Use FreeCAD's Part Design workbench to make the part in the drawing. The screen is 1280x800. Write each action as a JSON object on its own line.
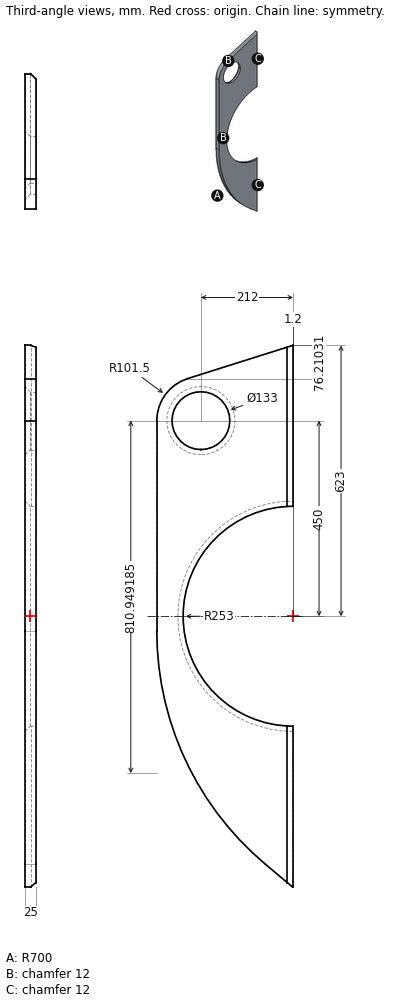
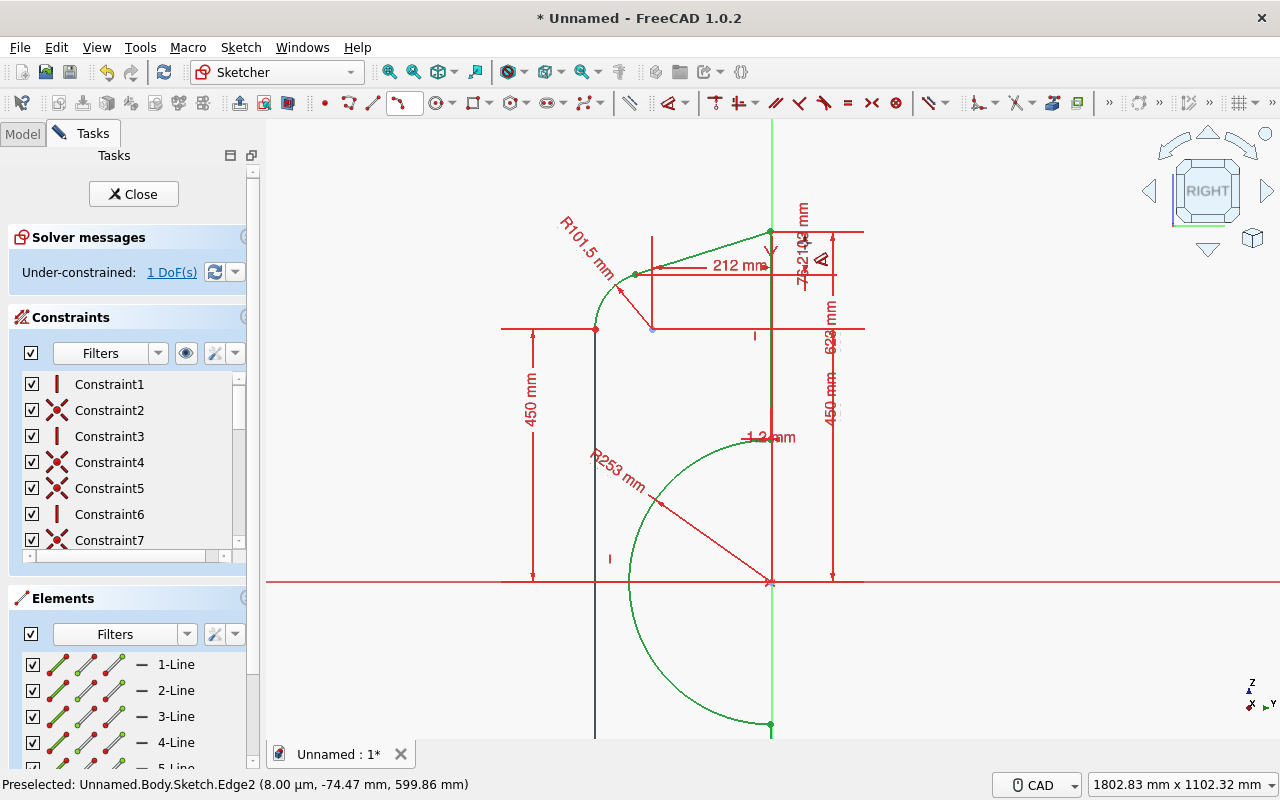
{"action": "left_click", "coordinate": [595, 467]}
{"action": "left_click", "coordinate": [561, 520]}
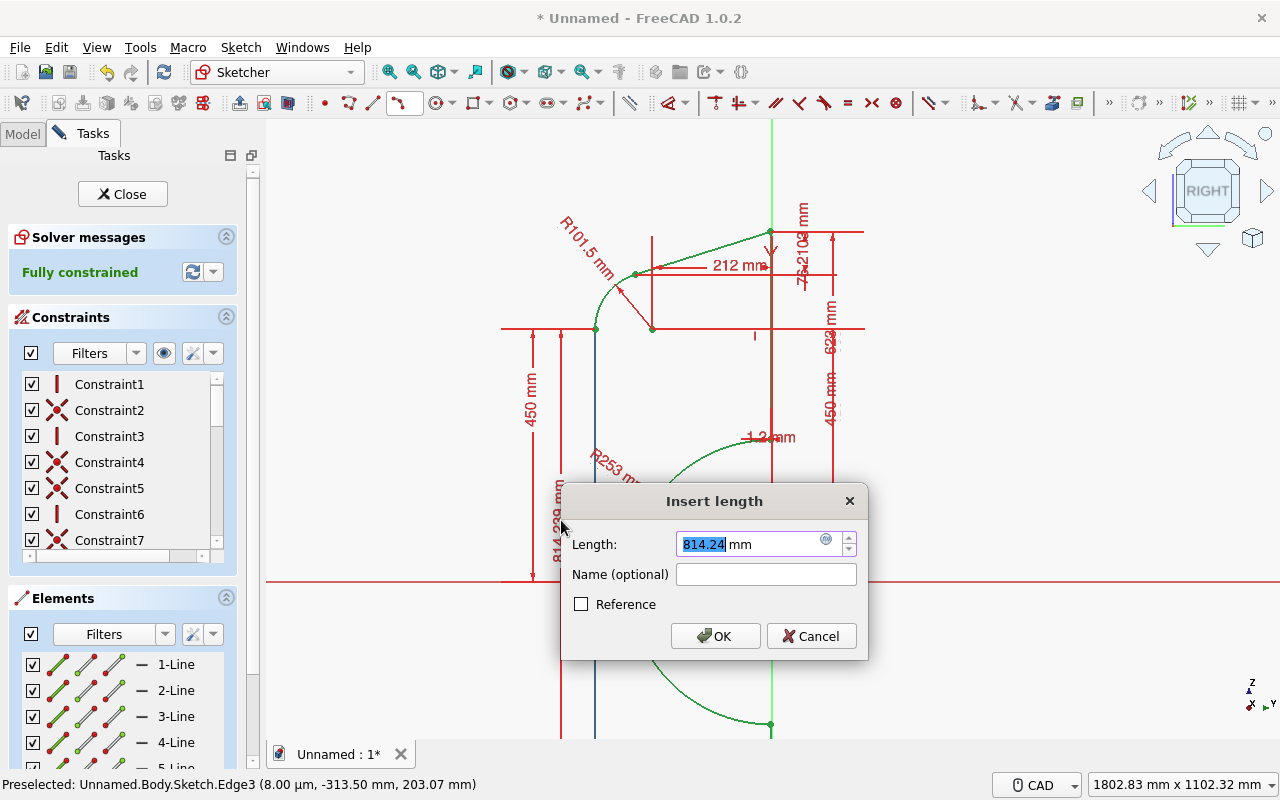
{"action": "type", "text": "810.949185"}
{"action": "key", "text": "Return"}
{"action": "key", "text": "Escape"}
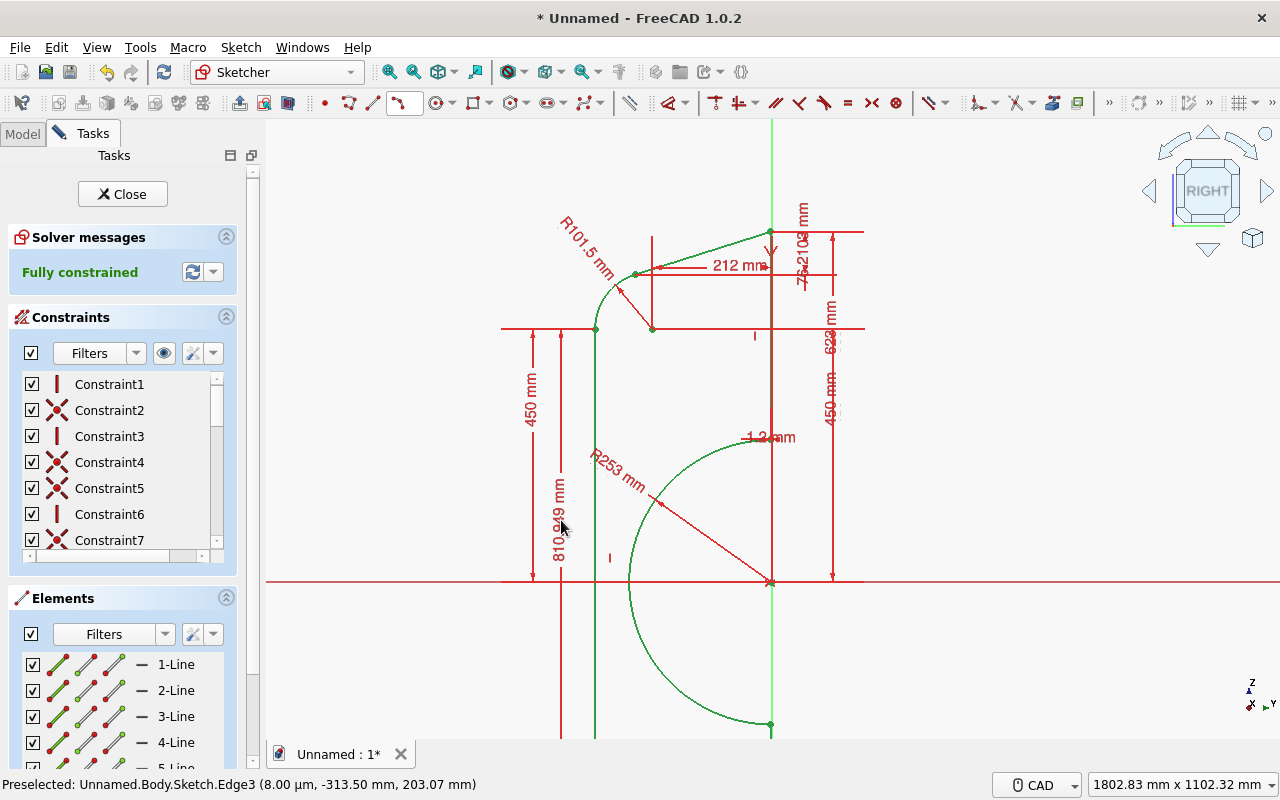
{"action": "left_click", "coordinate": [123, 194]}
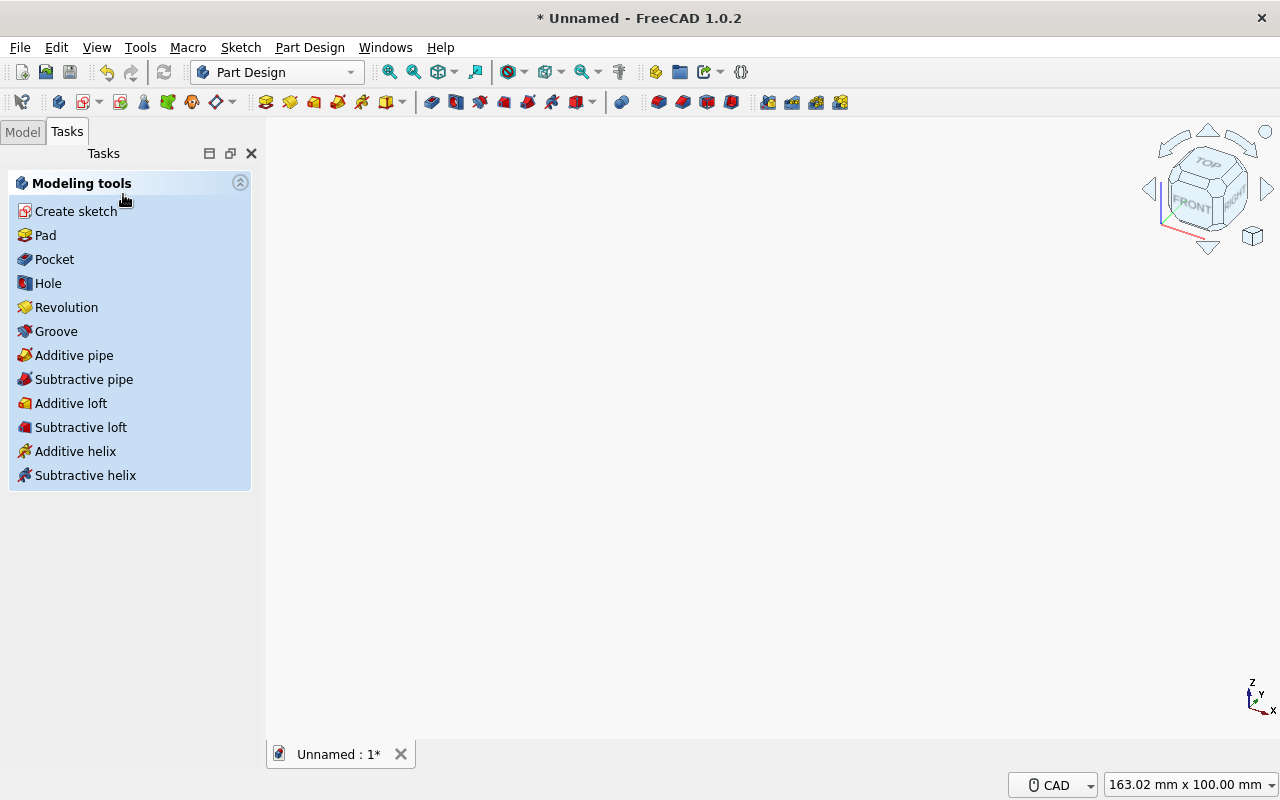
{"action": "left_click", "coordinate": [266, 102]}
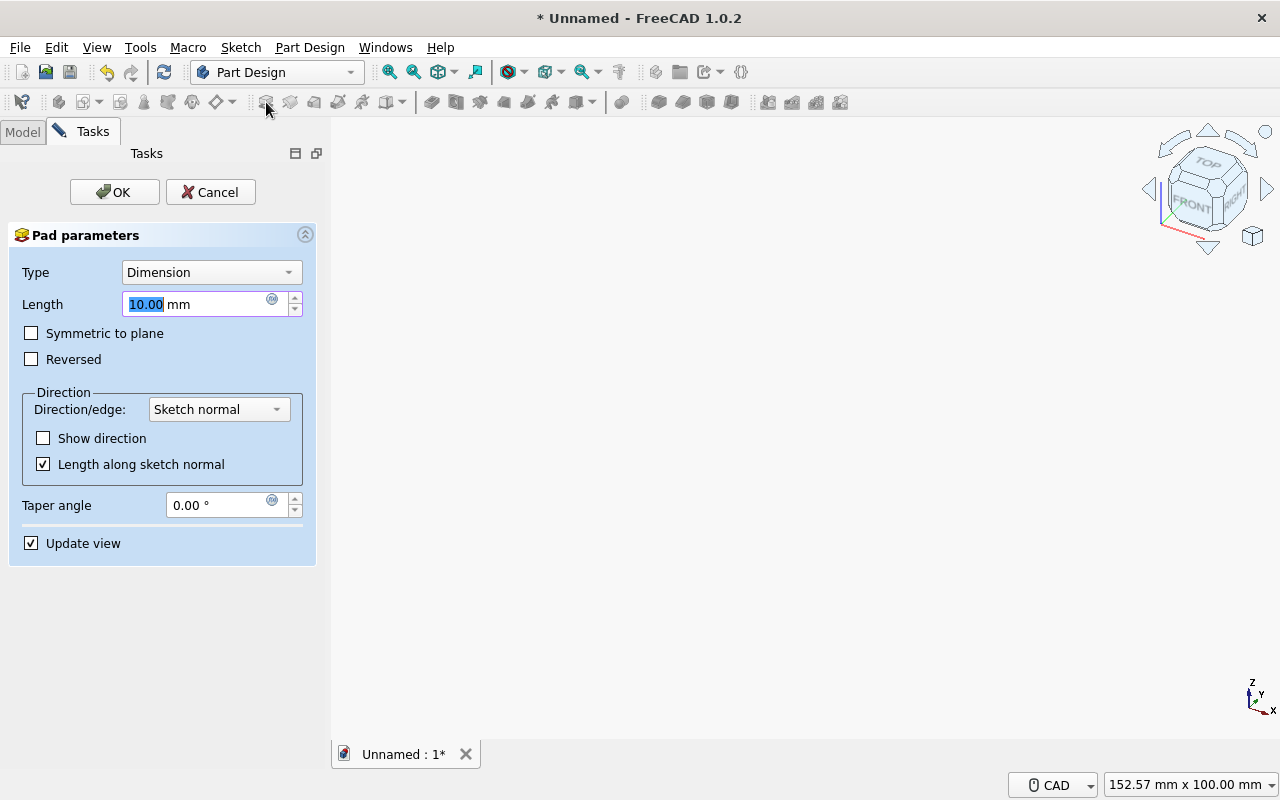
{"action": "type", "text": "25"}
{"action": "key", "text": "Tab"}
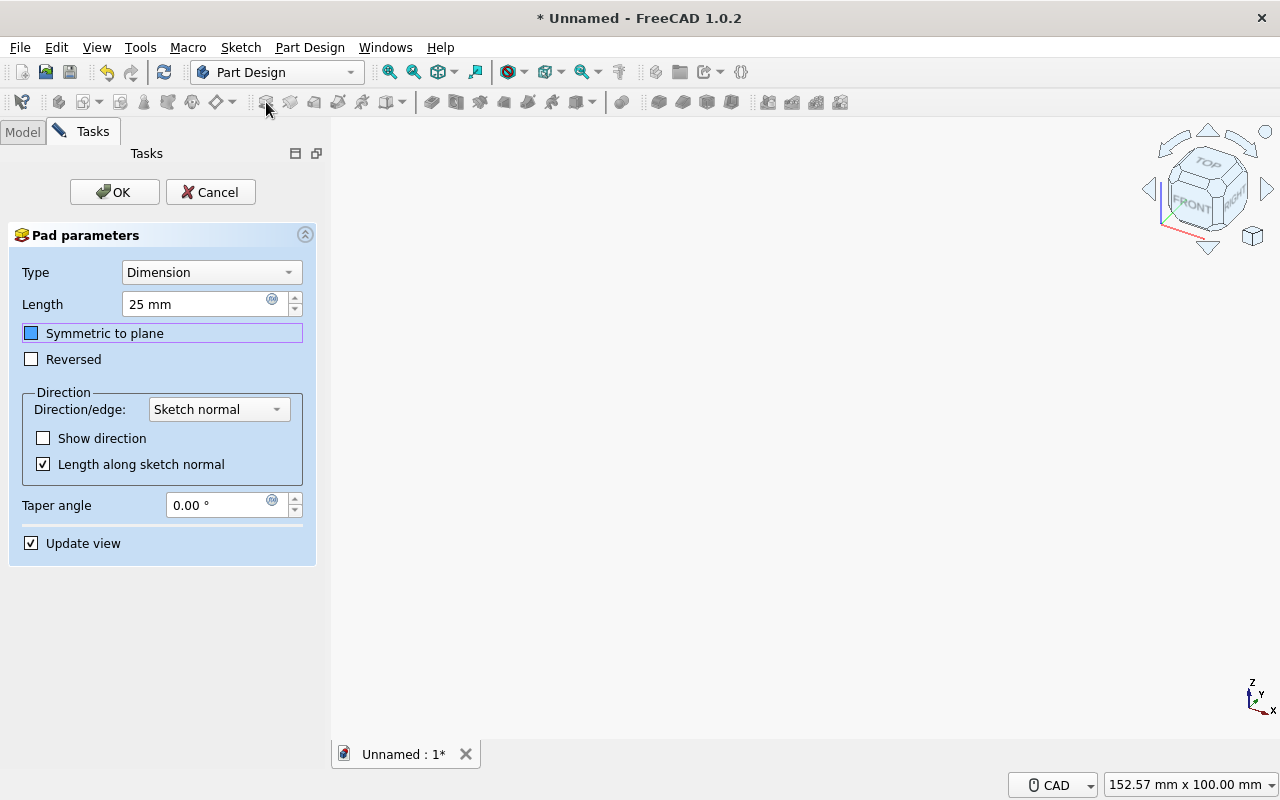
{"action": "left_click", "coordinate": [30, 333]}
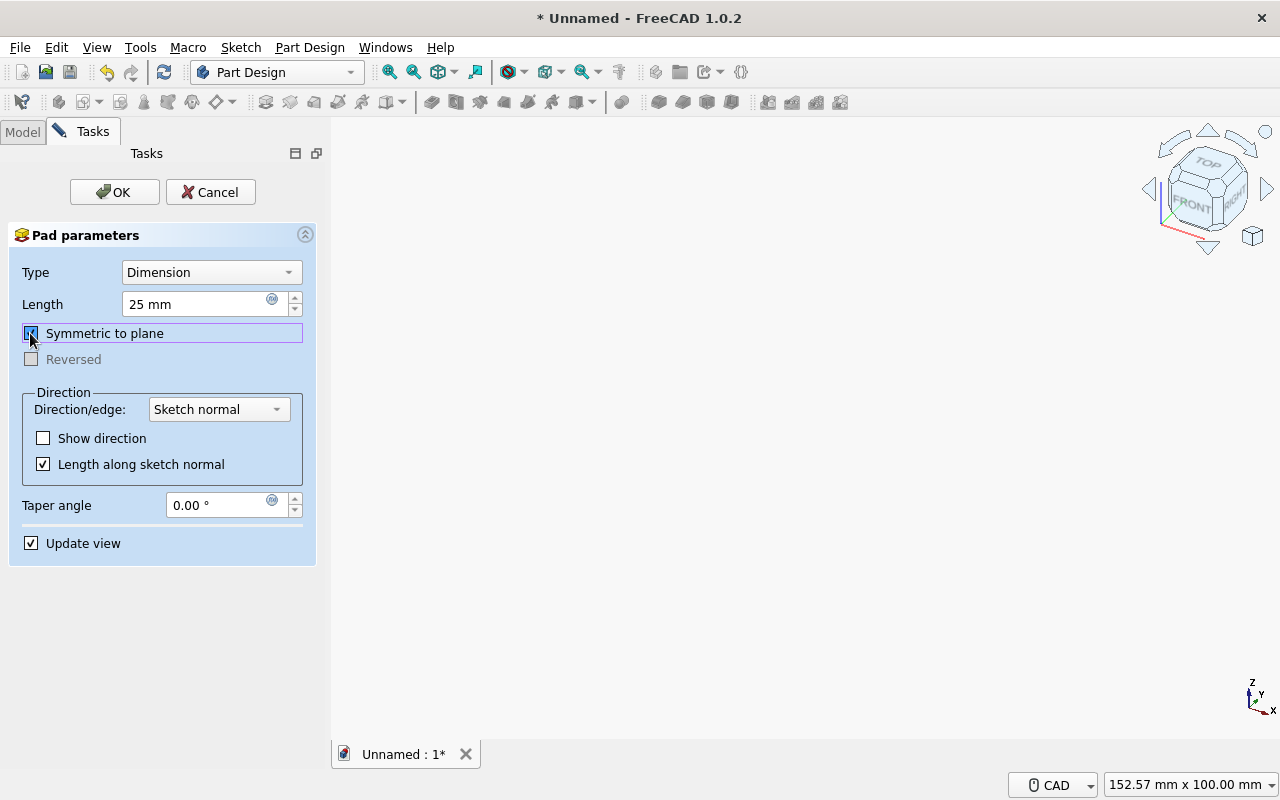
{"action": "left_click", "coordinate": [115, 192]}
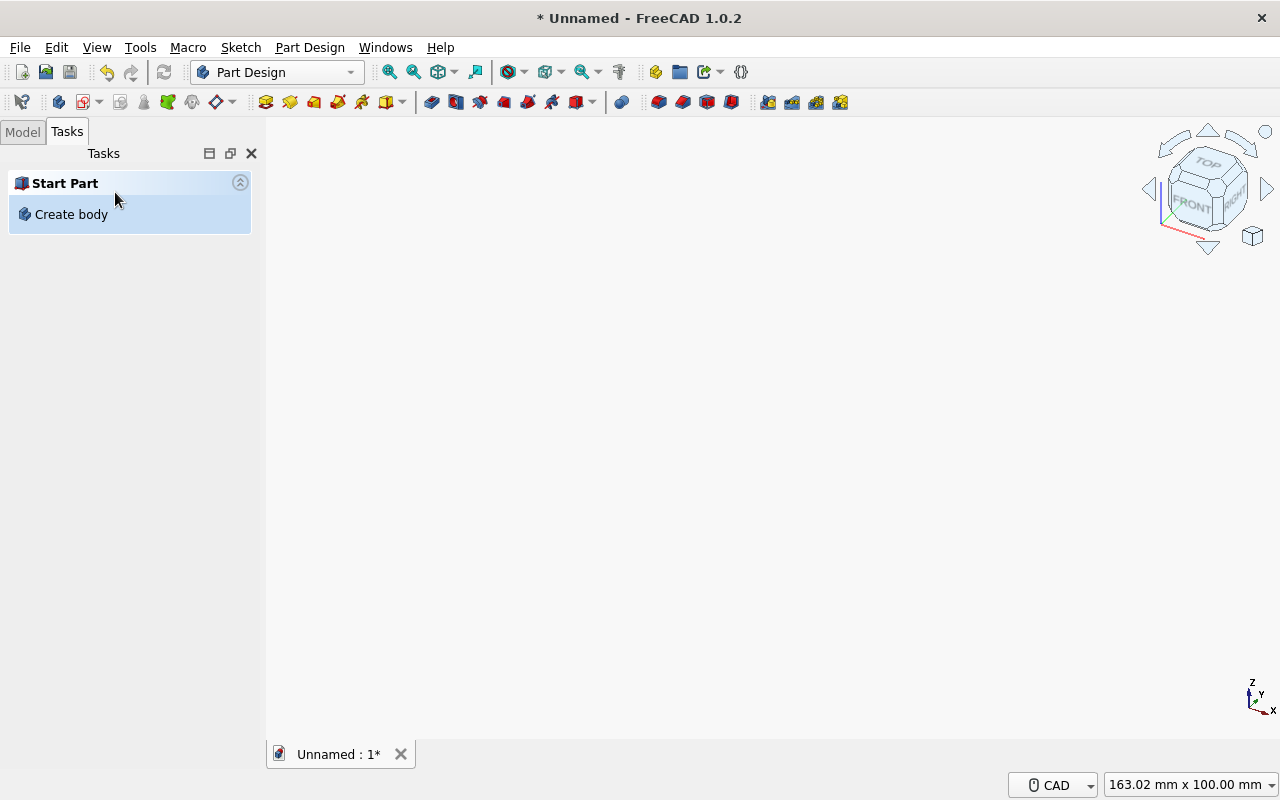
{"action": "left_click", "coordinate": [390, 72]}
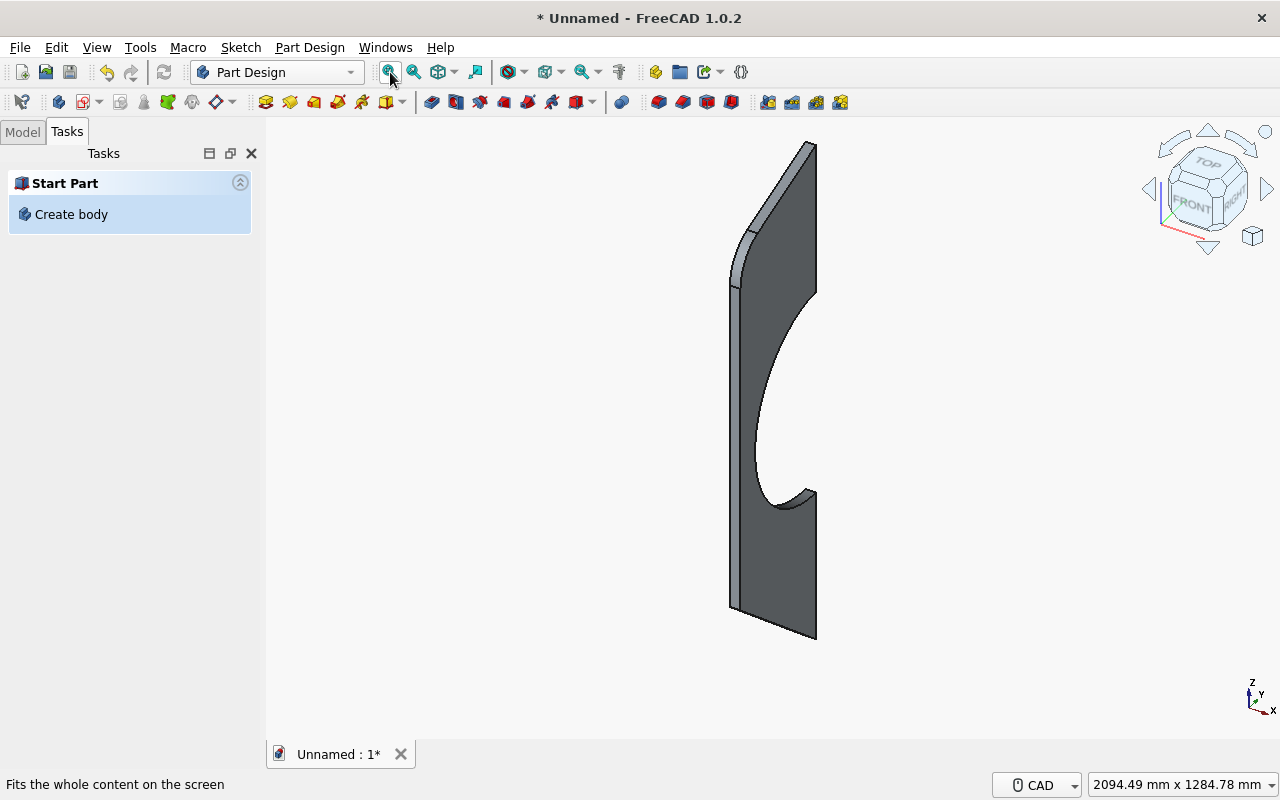
{"action": "left_click", "coordinate": [84, 102]}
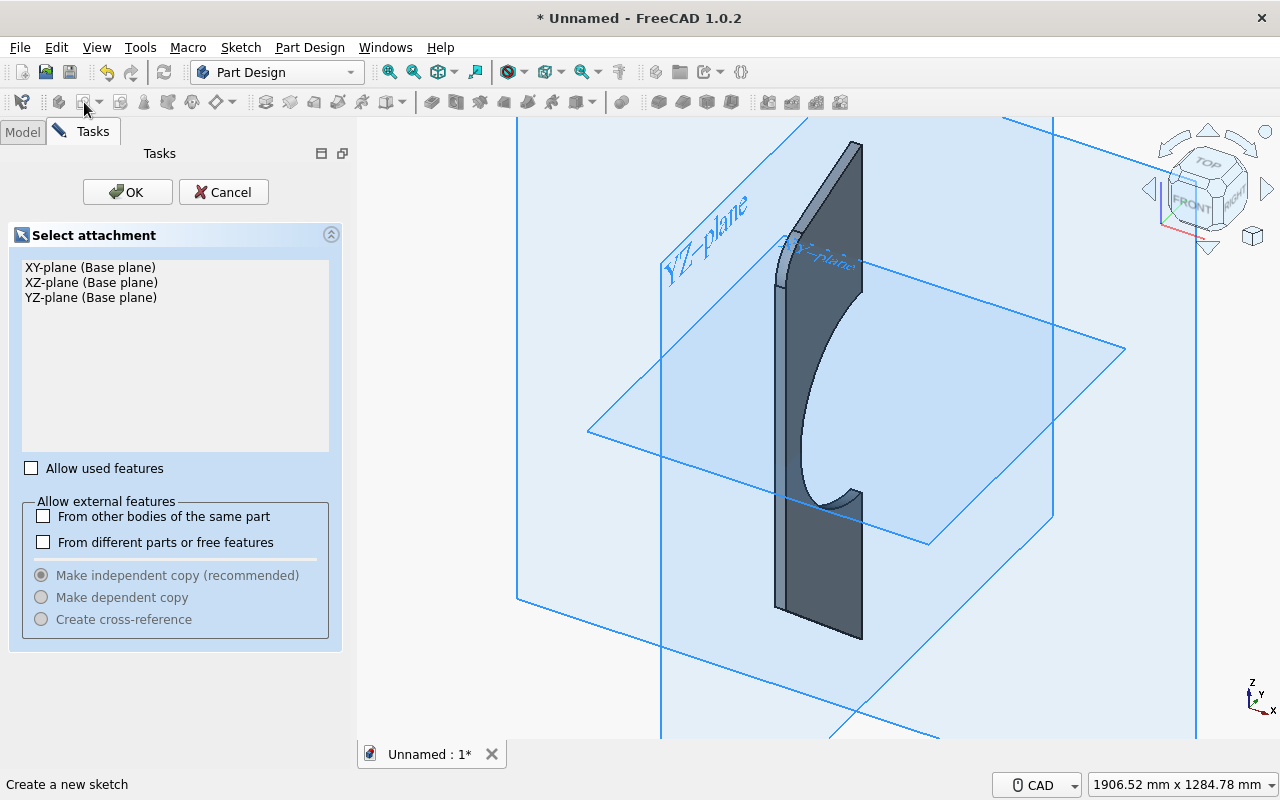
{"action": "left_click", "coordinate": [82, 298]}